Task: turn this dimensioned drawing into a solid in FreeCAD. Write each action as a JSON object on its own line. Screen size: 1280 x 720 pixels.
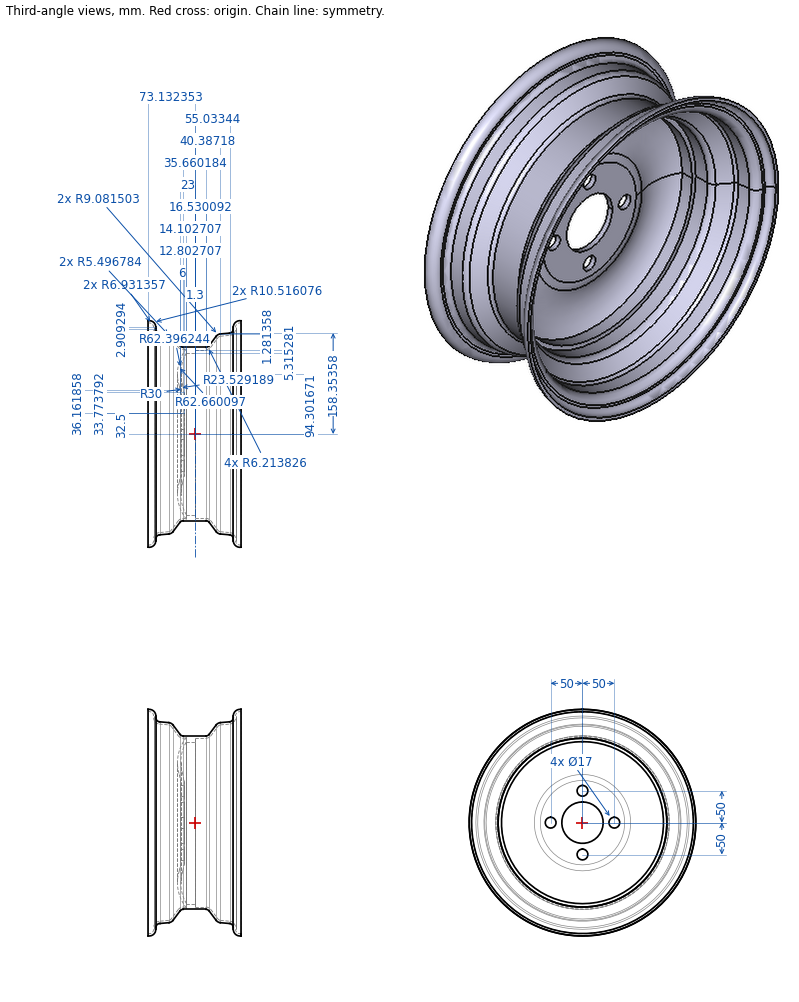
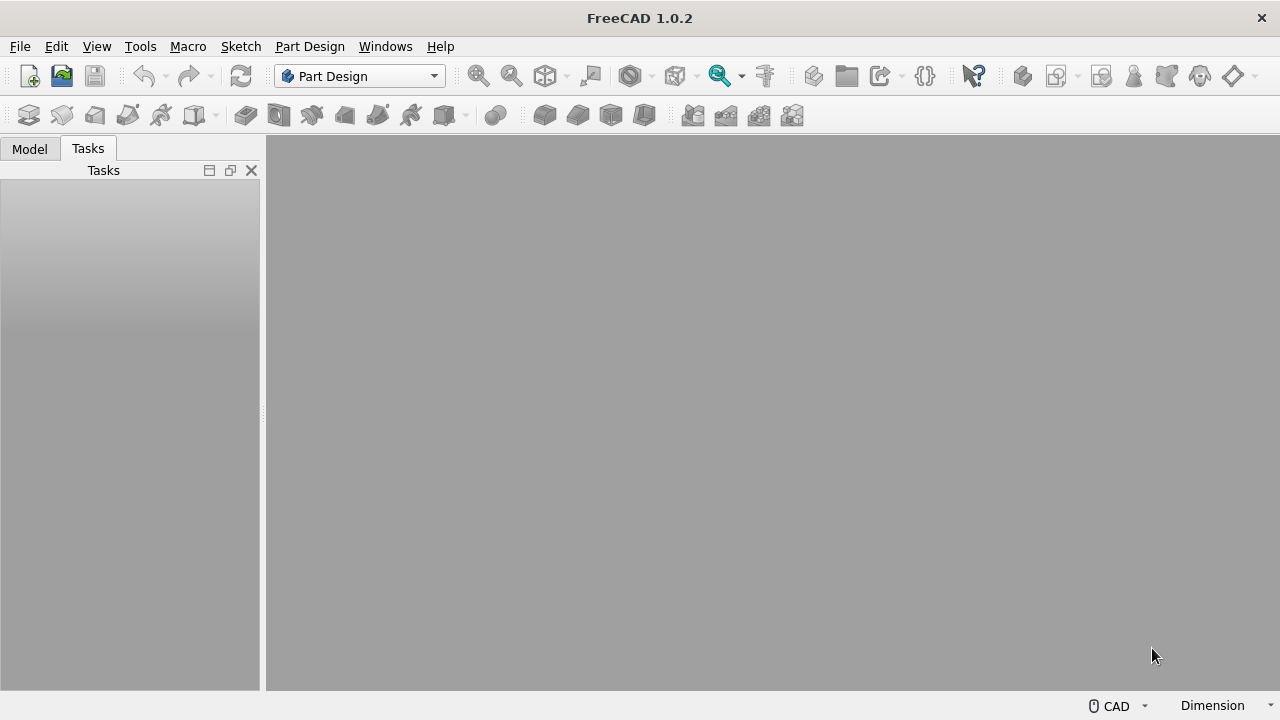
{"action": "key", "text": "ctrl+n"}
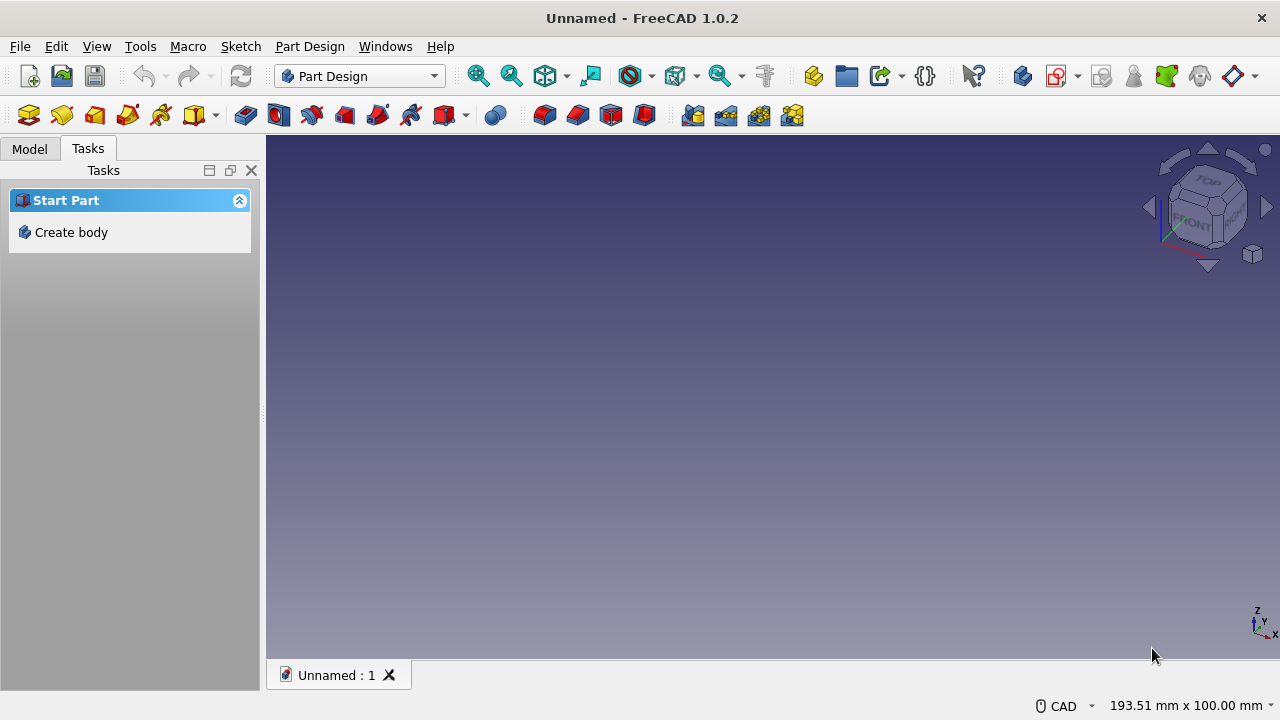
{"action": "left_click", "coordinate": [1056, 76]}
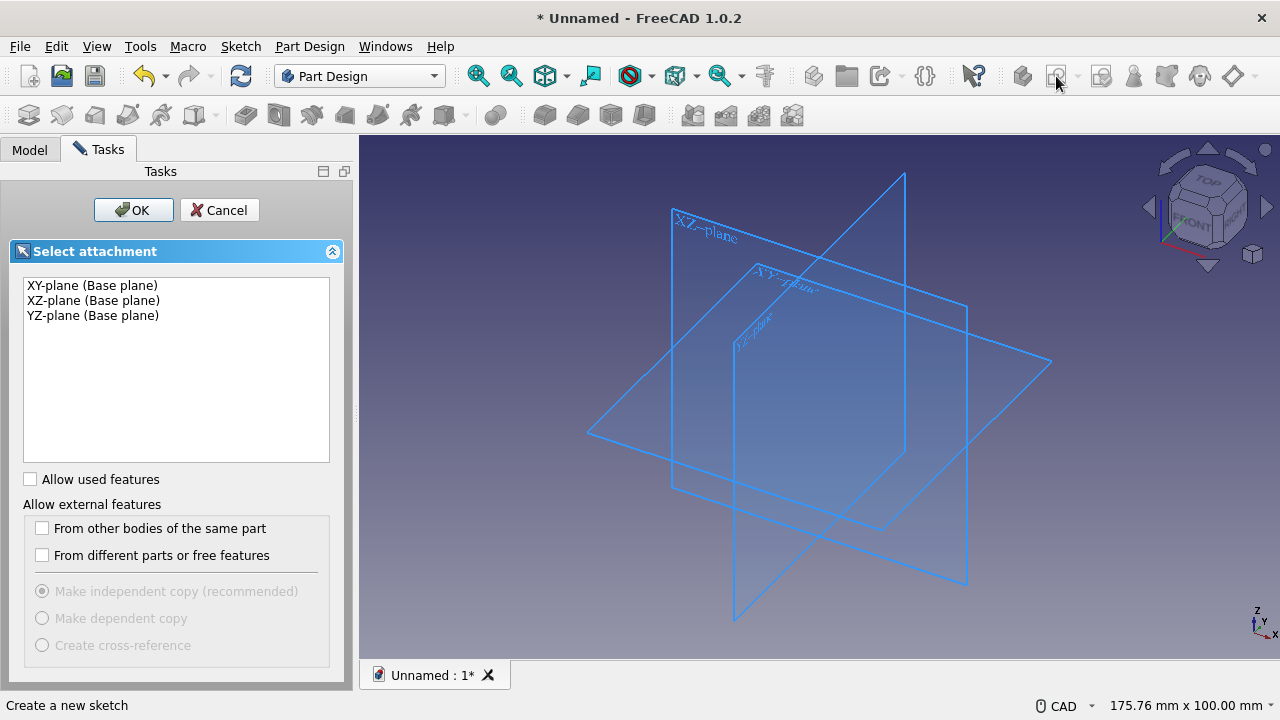
{"action": "left_click", "coordinate": [84, 286]}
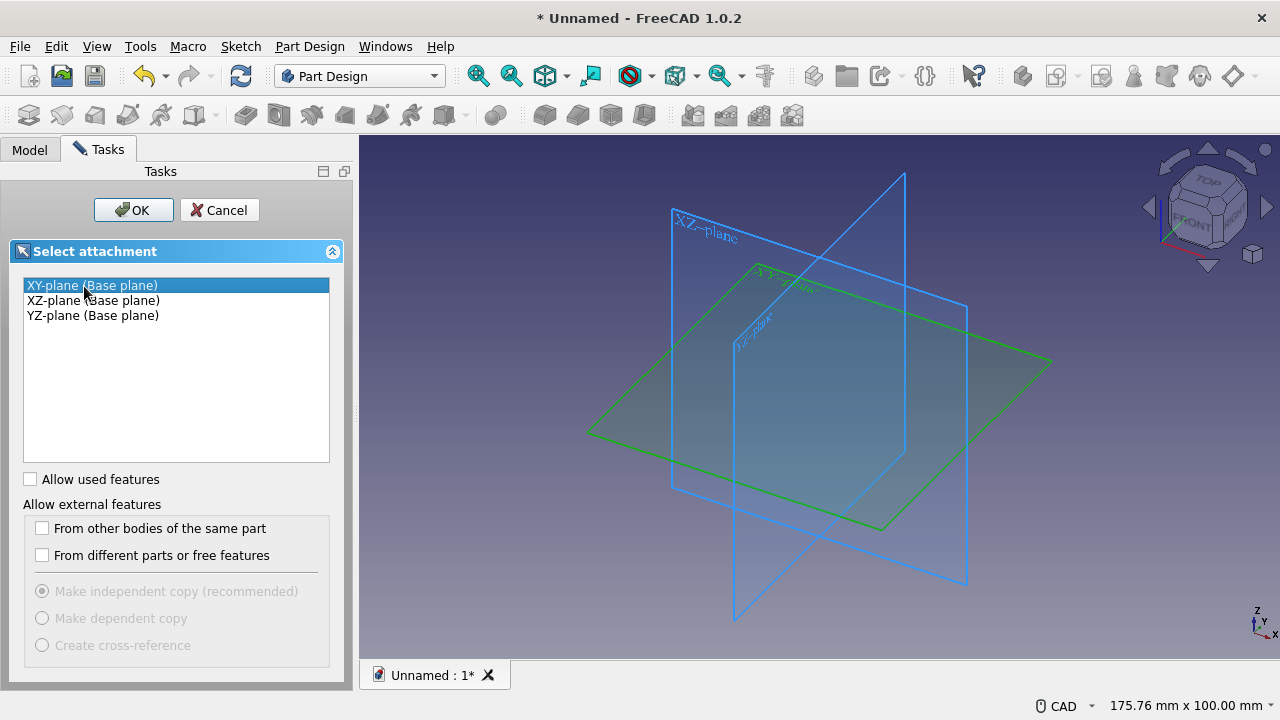
{"action": "left_click", "coordinate": [134, 210]}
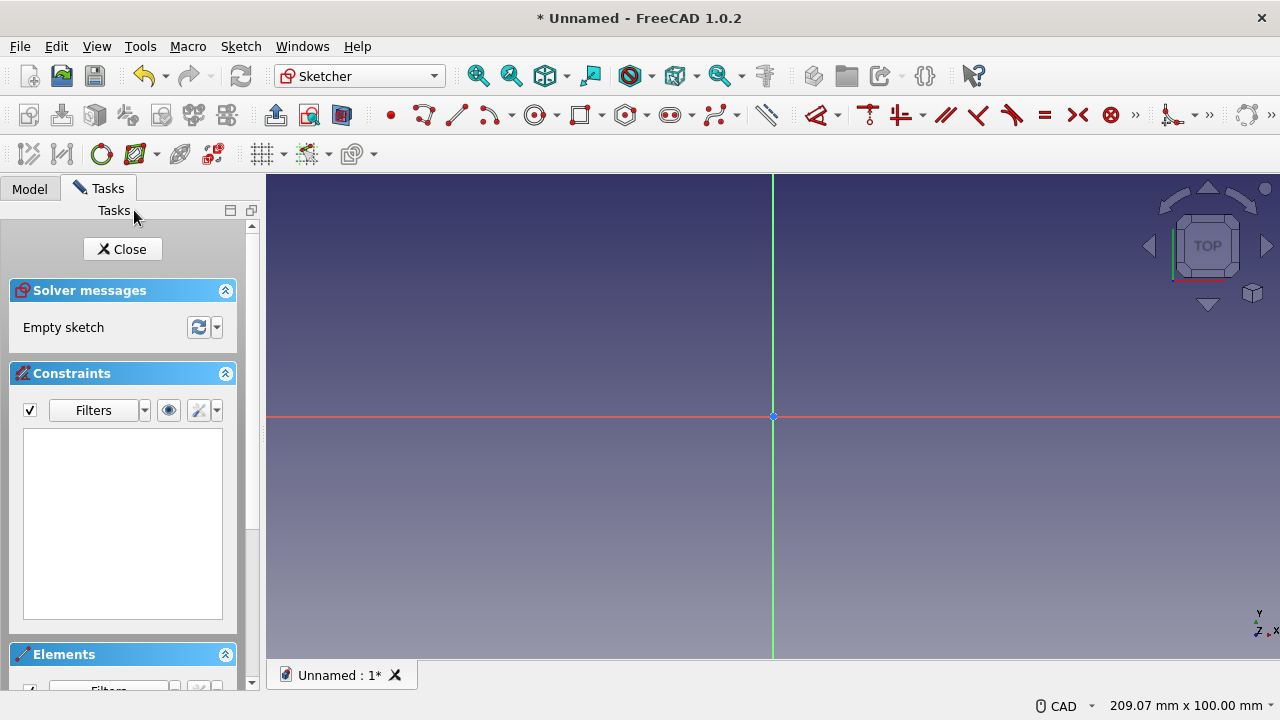
{"action": "scroll", "coordinate": [665, 631], "scroll_direction": "down", "scroll_amount": 5}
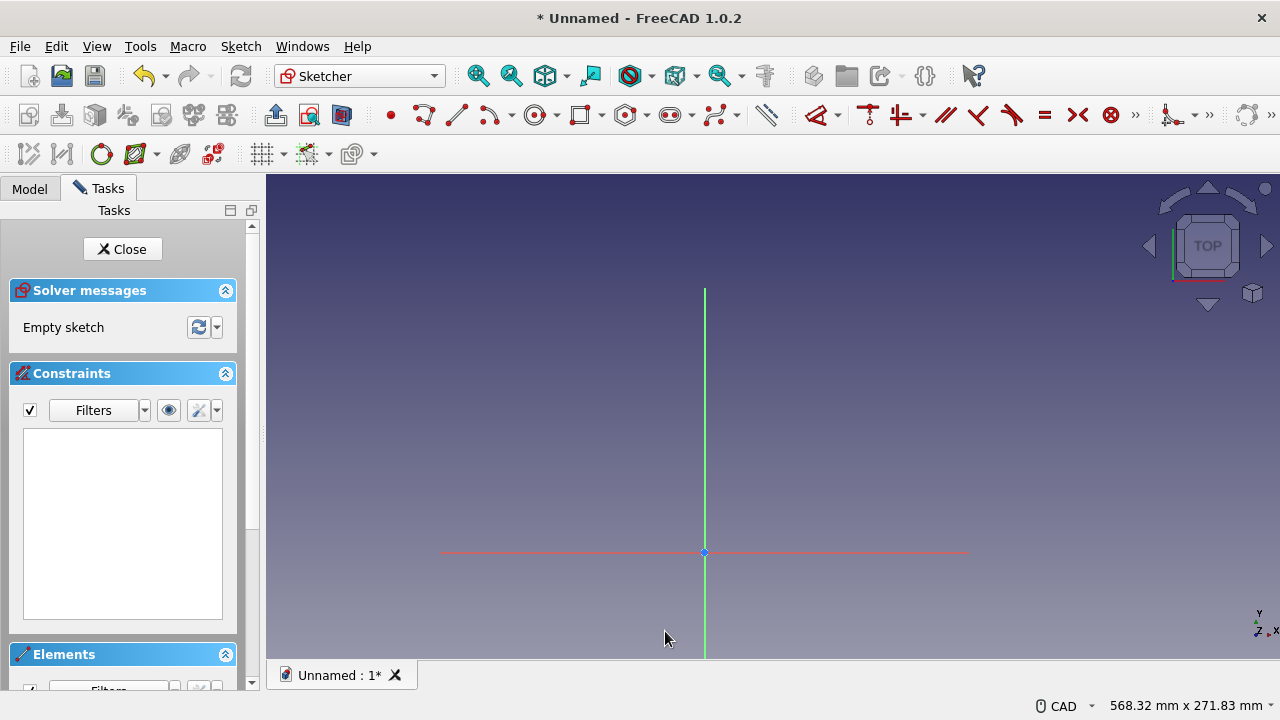
{"action": "key", "text": "g l"}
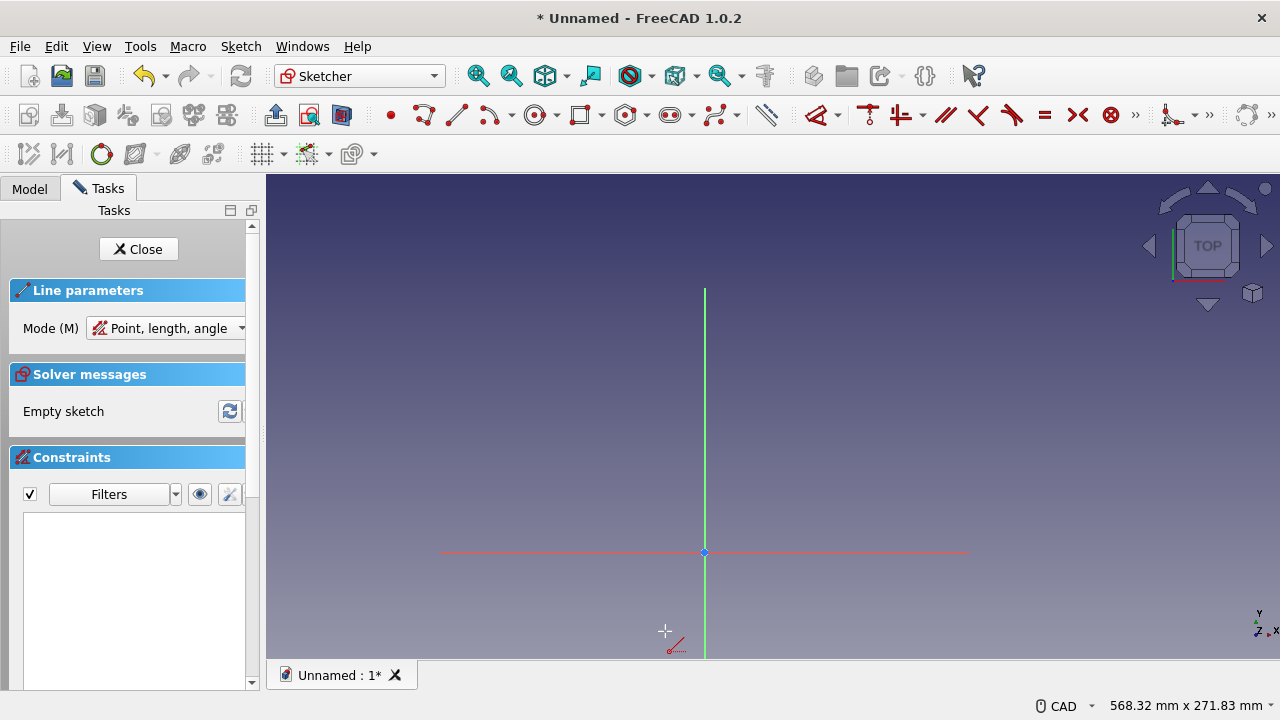
{"action": "left_click", "coordinate": [803, 270]}
{"action": "left_click", "coordinate": [777, 273]}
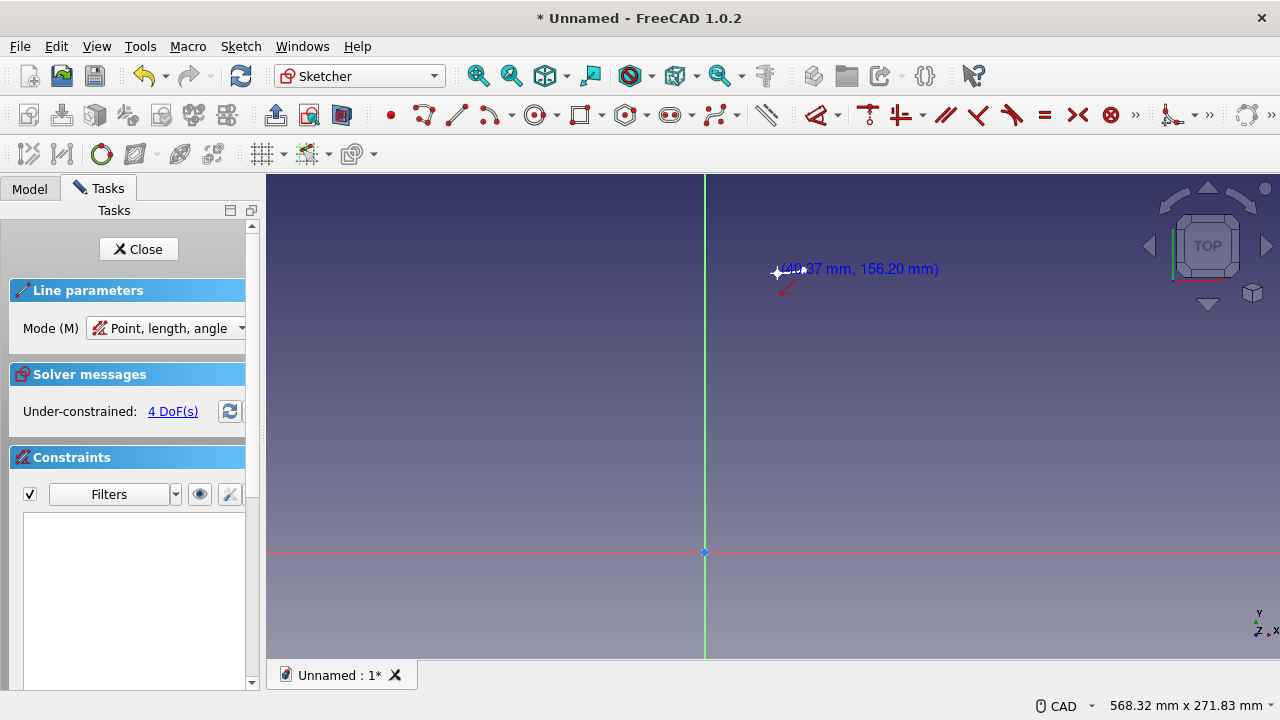
{"action": "left_click", "coordinate": [765, 279]}
{"action": "left_click", "coordinate": [746, 305]}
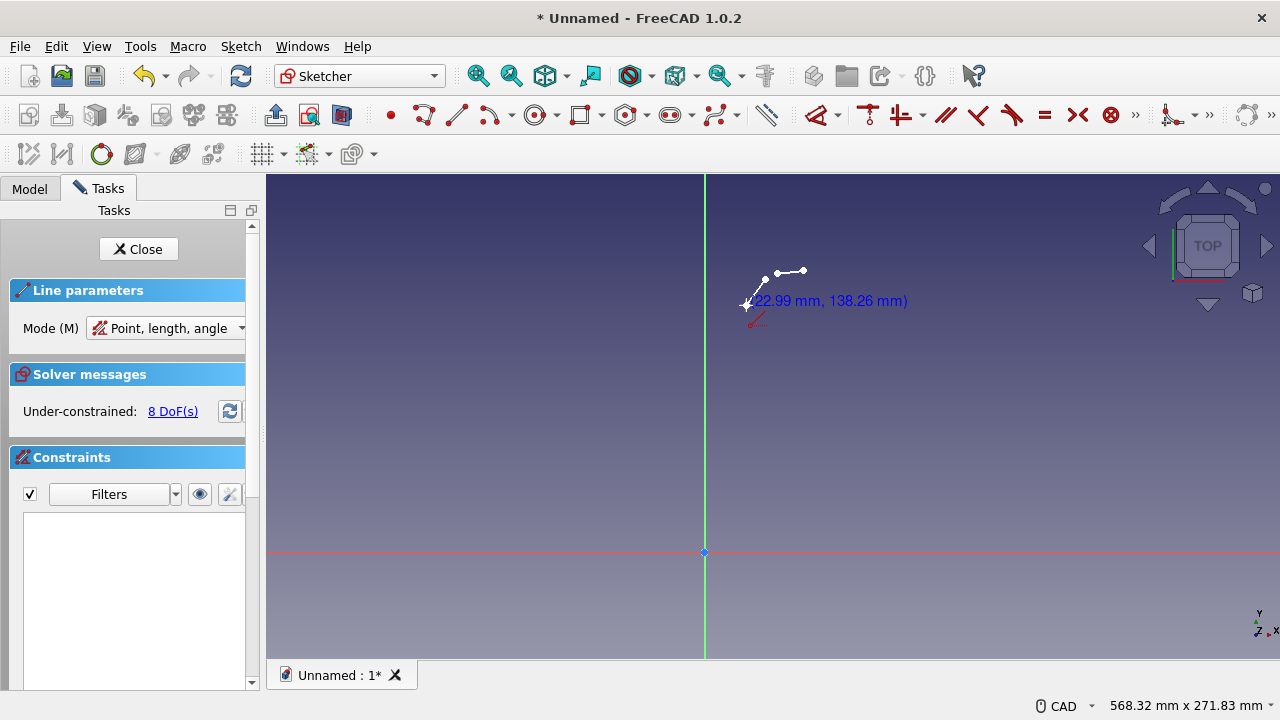
{"action": "scroll", "coordinate": [737, 310], "scroll_direction": "up", "scroll_amount": 3}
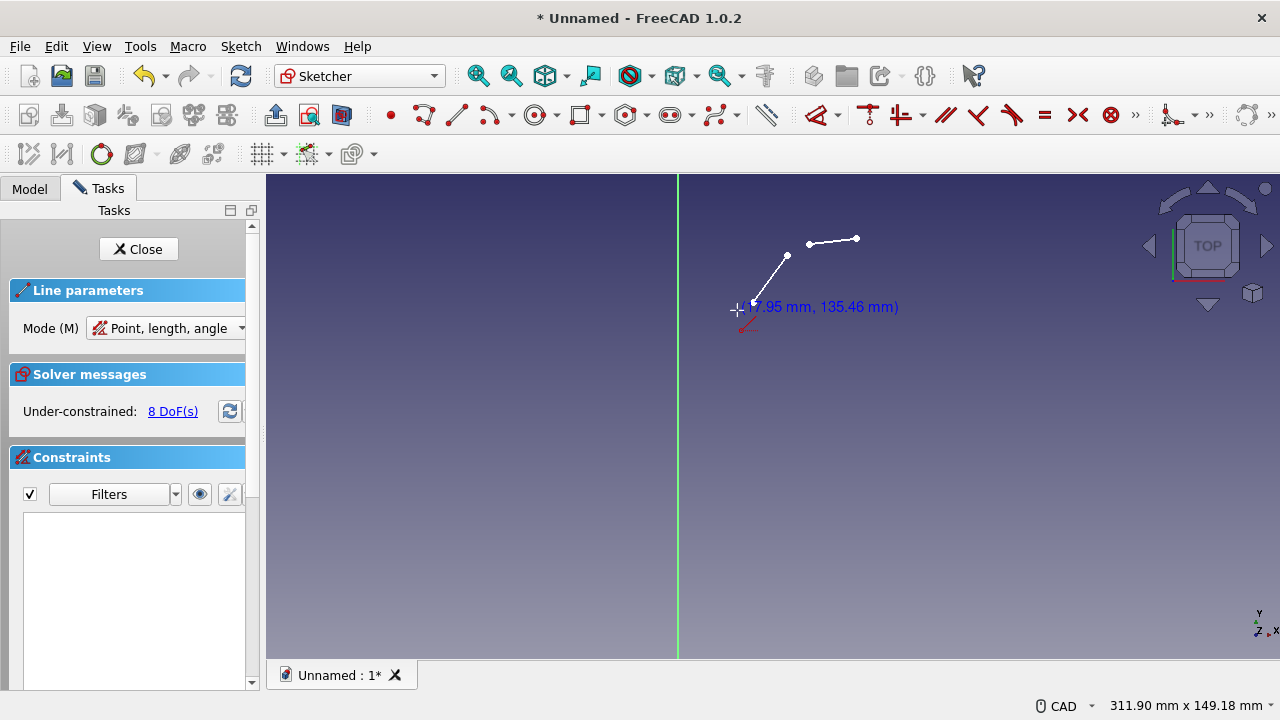
{"action": "left_click", "coordinate": [736, 310]}
{"action": "left_click", "coordinate": [620, 310]}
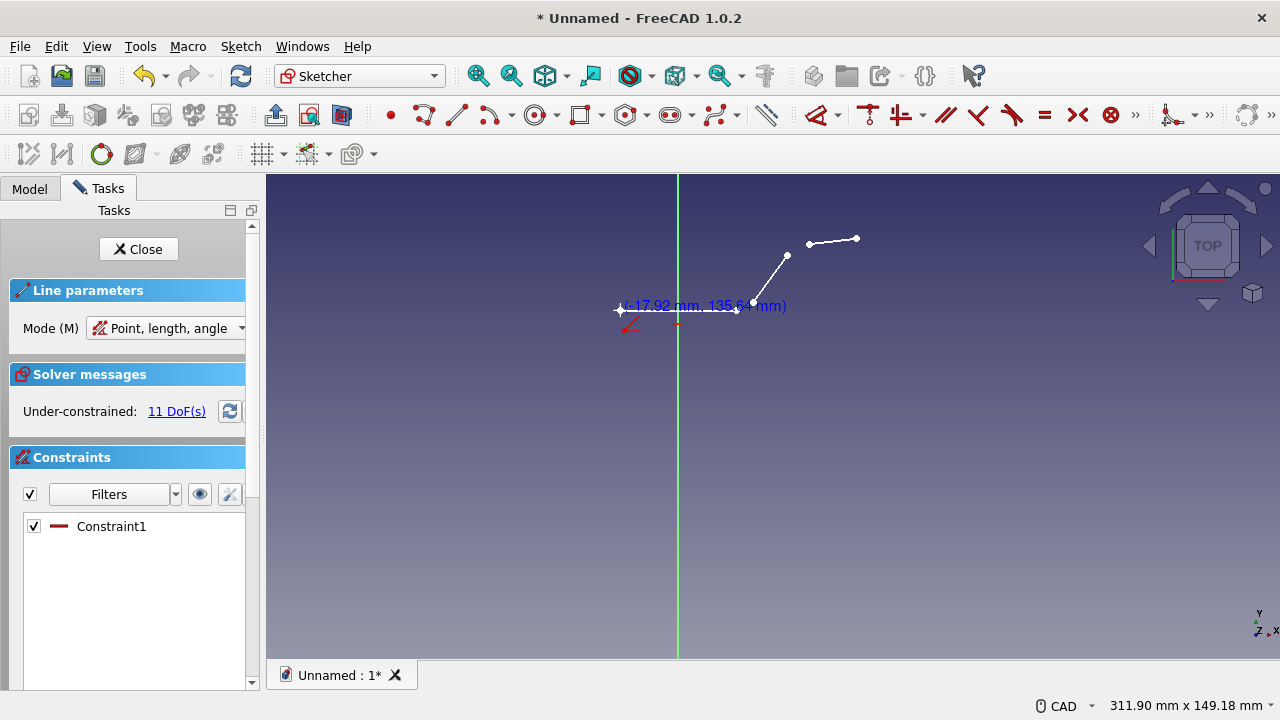
{"action": "left_click", "coordinate": [604, 301]}
{"action": "left_click", "coordinate": [568, 253]}